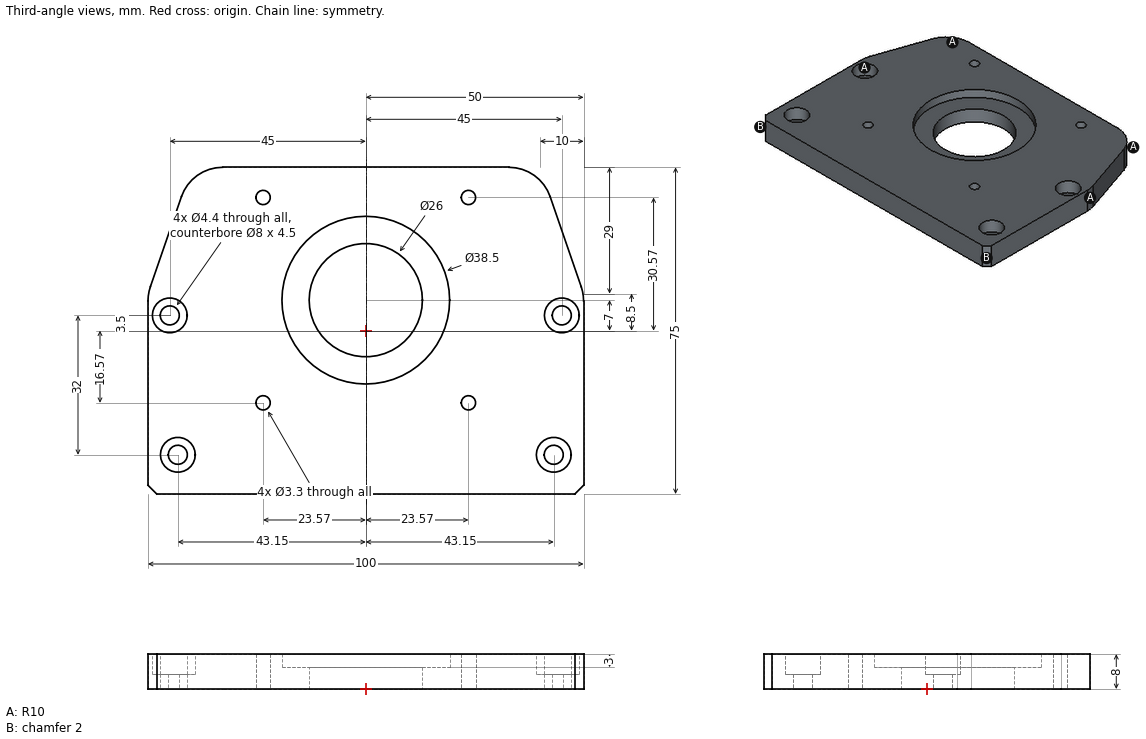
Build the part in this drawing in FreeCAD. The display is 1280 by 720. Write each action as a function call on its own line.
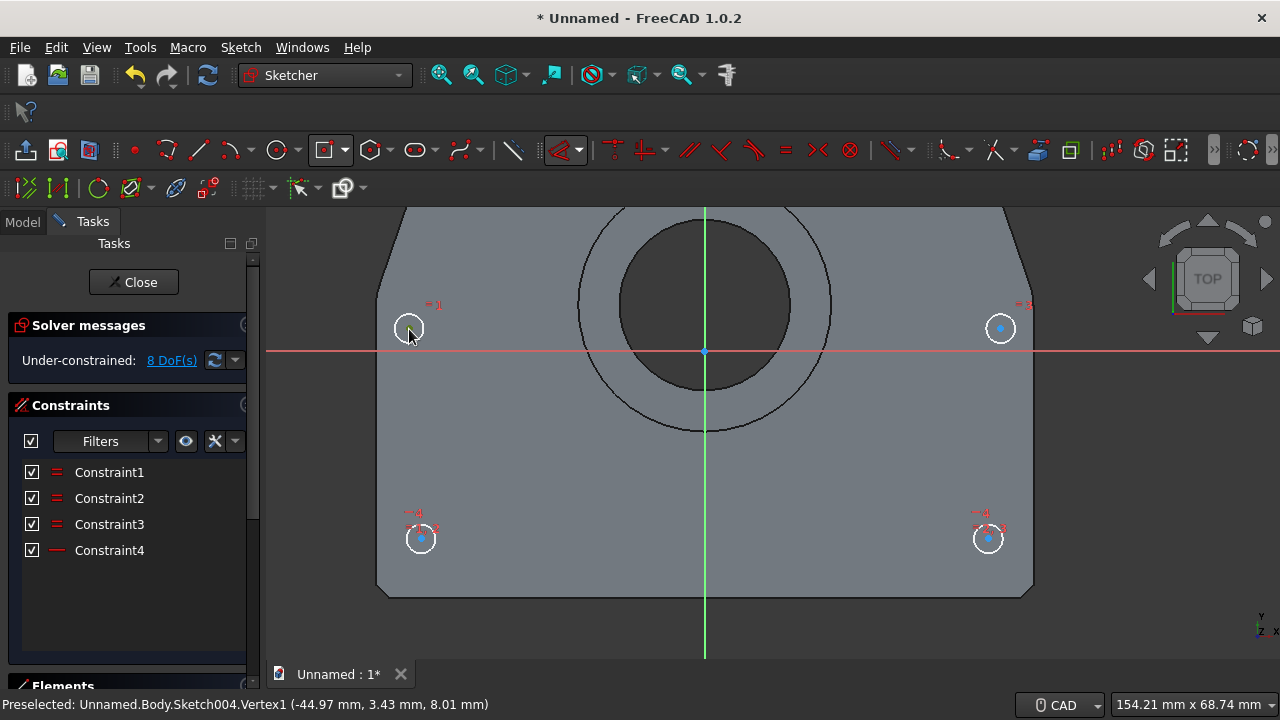
click(1001, 329)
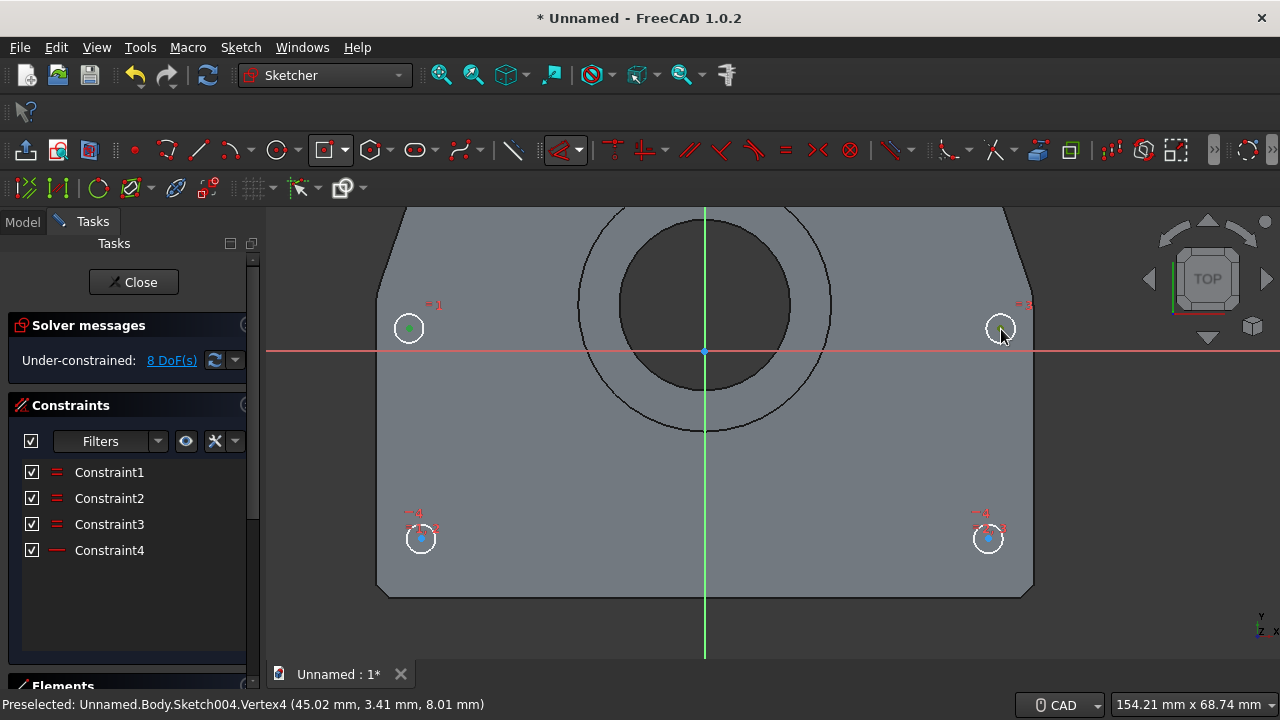
click(668, 150)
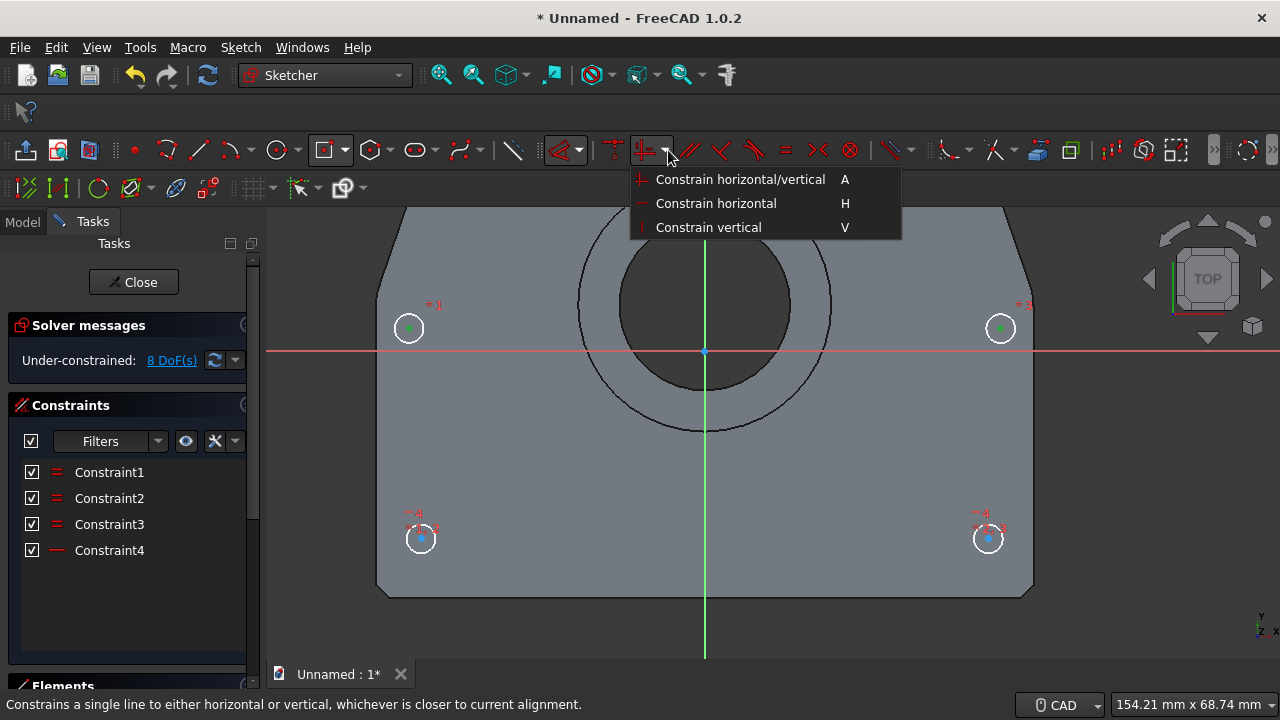
click(766, 203)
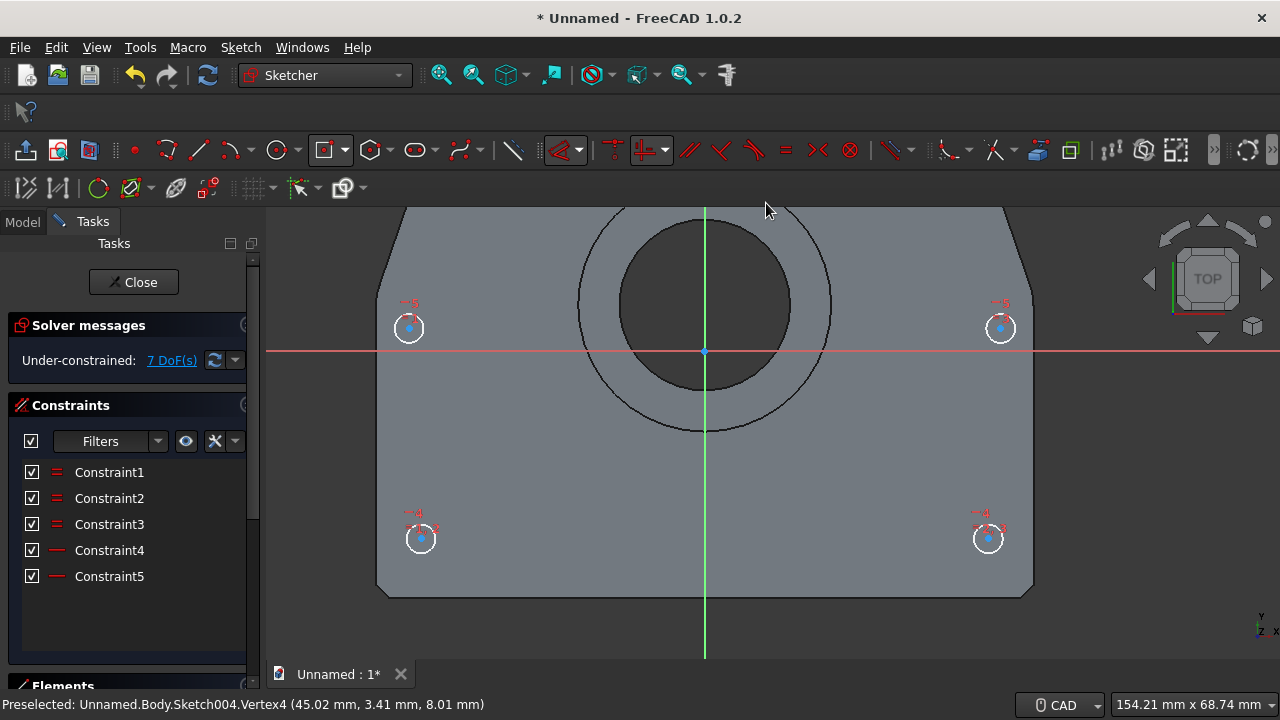
scroll(419, 318, up, 2)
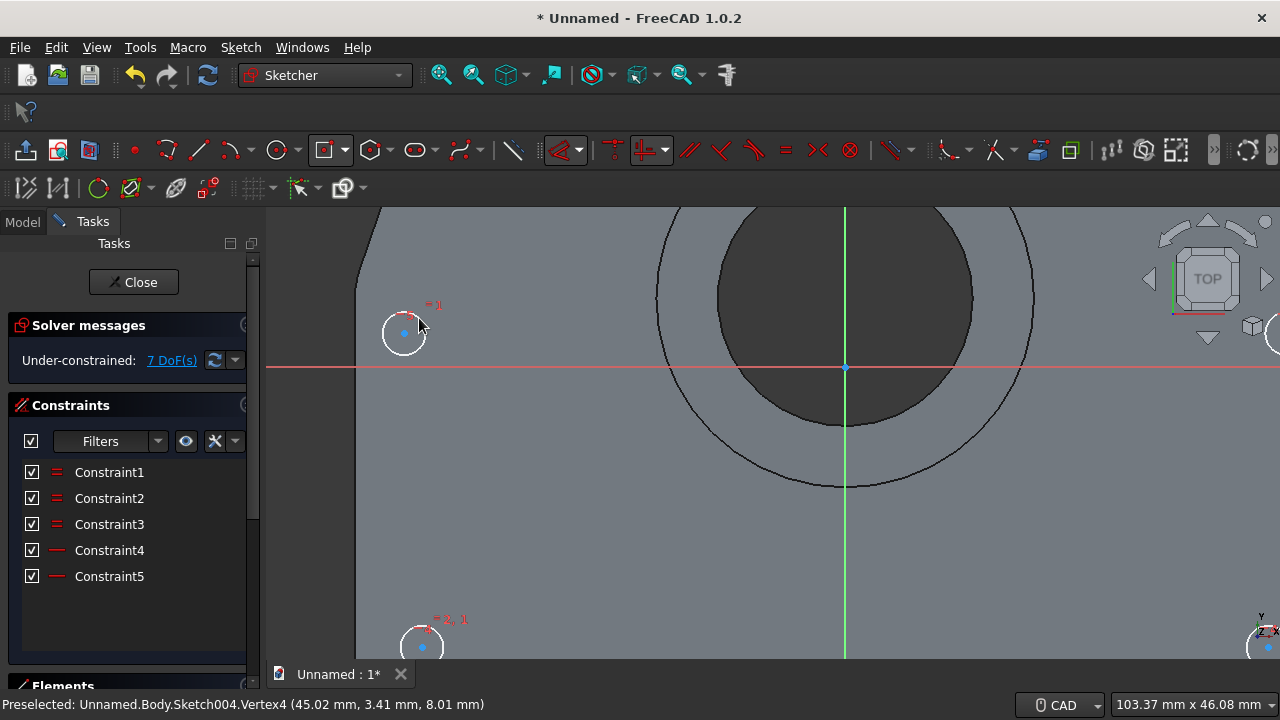
click(419, 318)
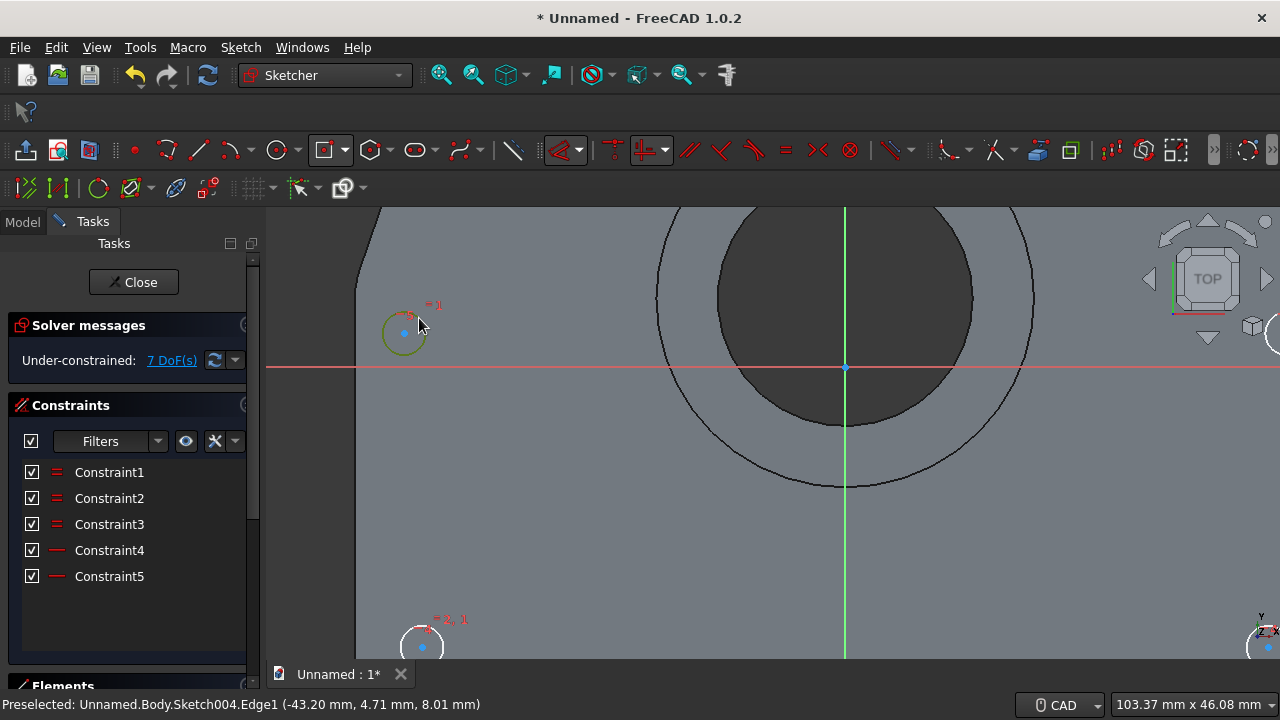
key(k)
key(o)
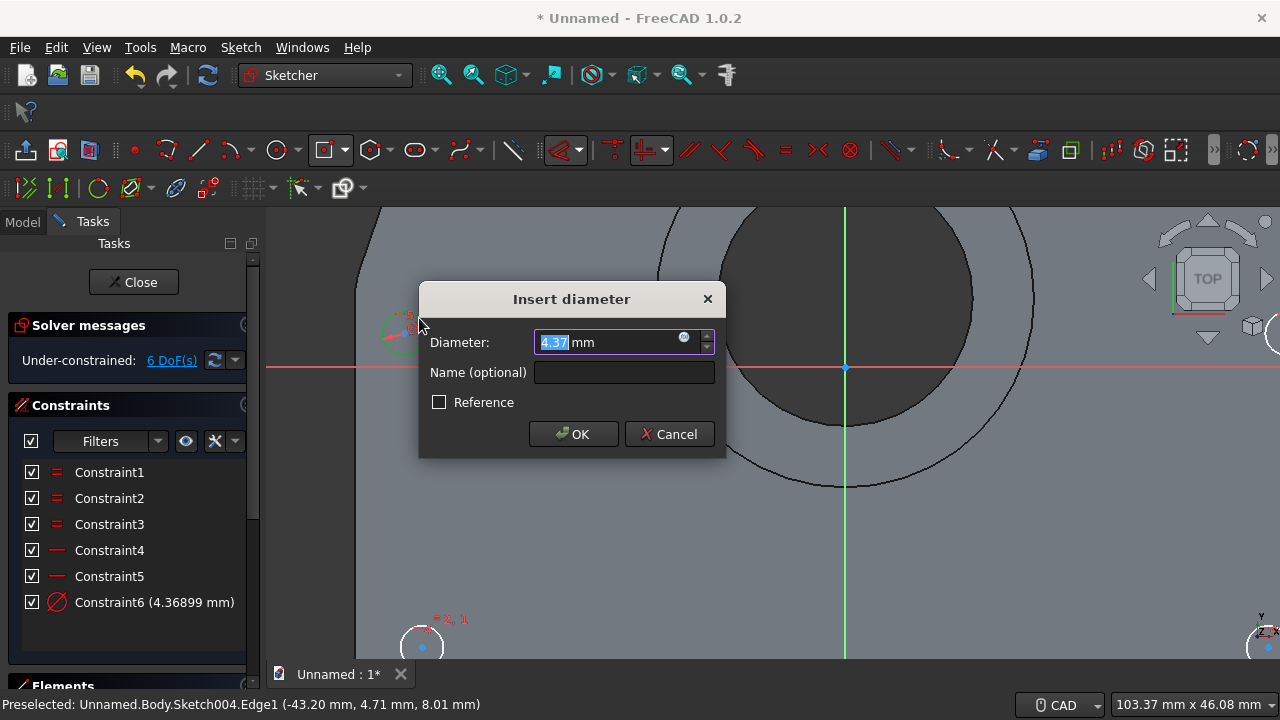
text(4.4)
key(Return)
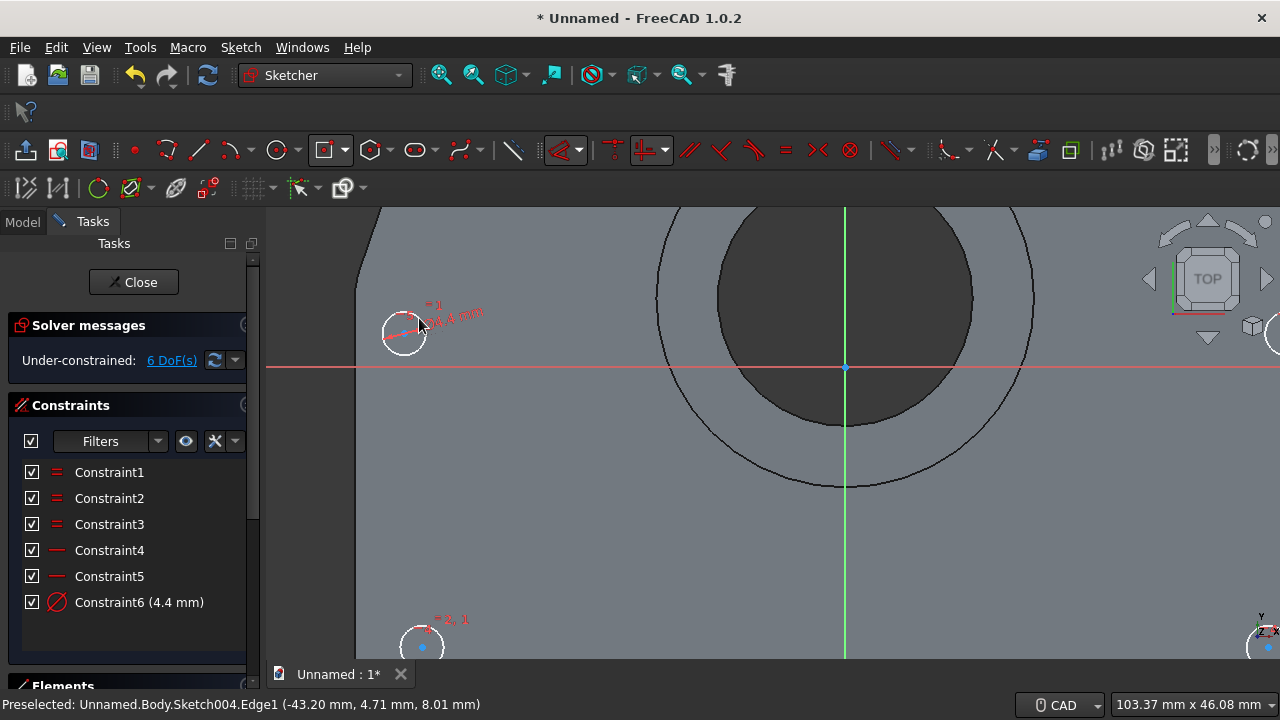
click(404, 334)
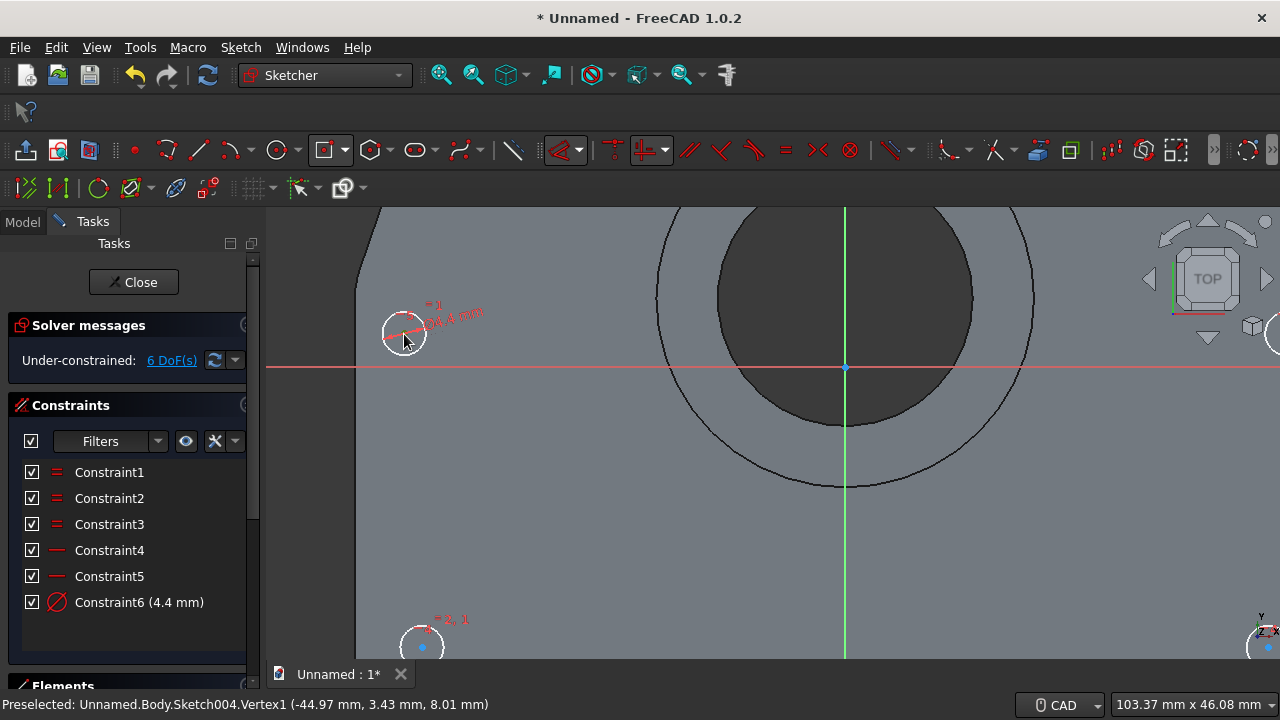
key(l)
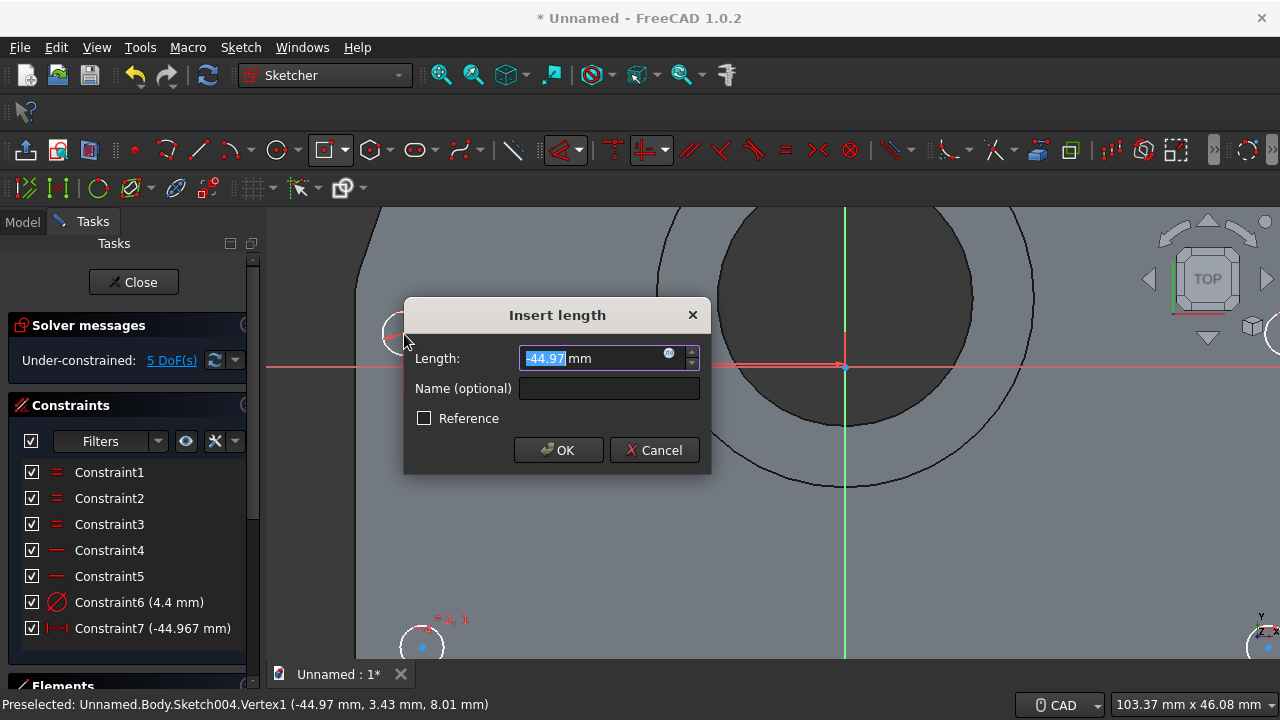
text(-45)
key(Return)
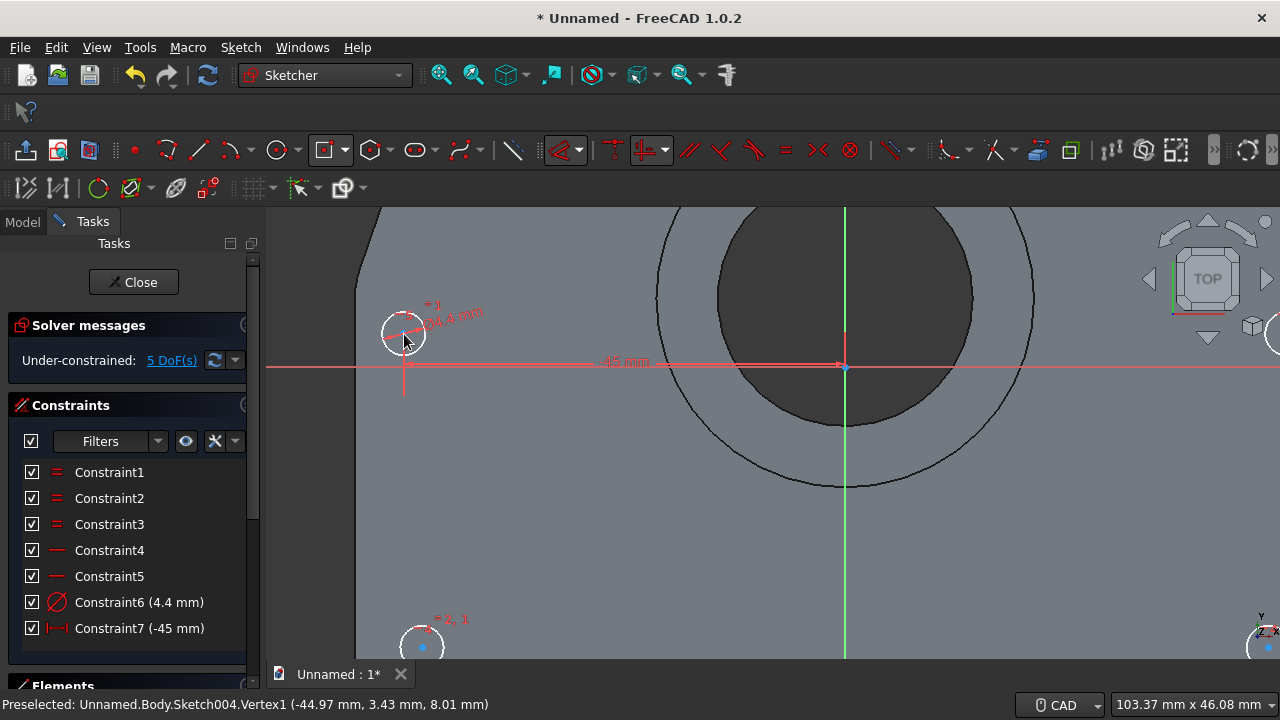
scroll(418, 317, down, 2)